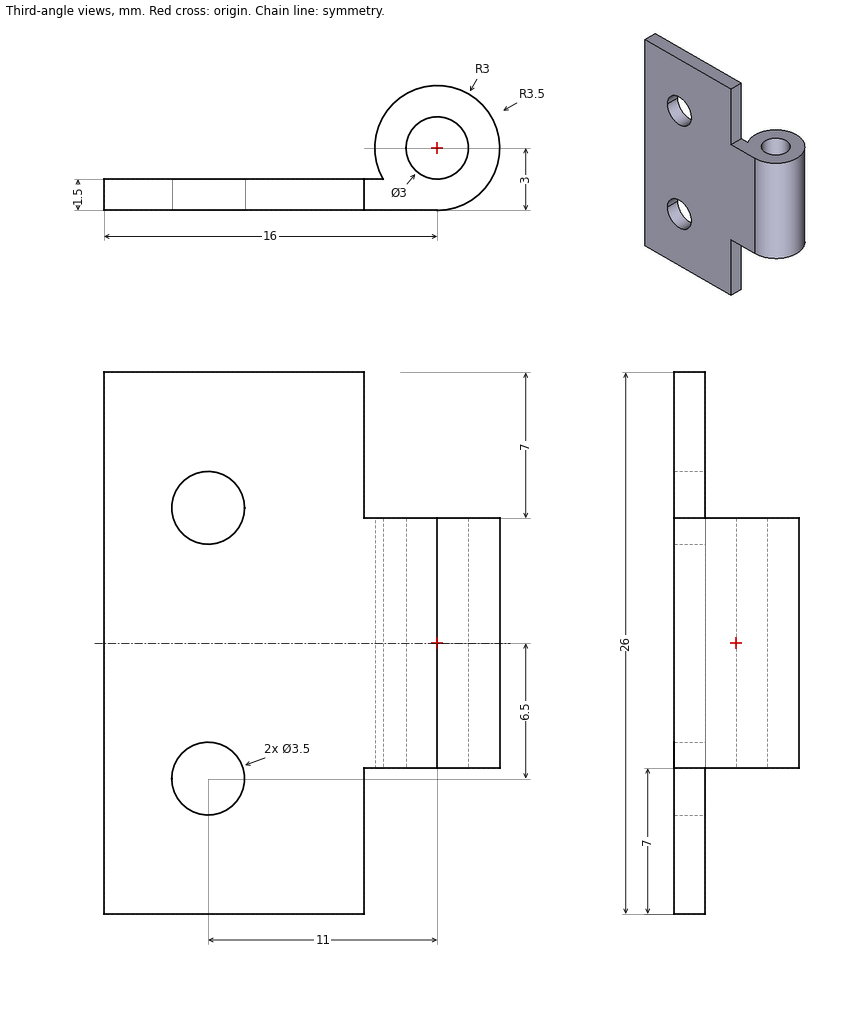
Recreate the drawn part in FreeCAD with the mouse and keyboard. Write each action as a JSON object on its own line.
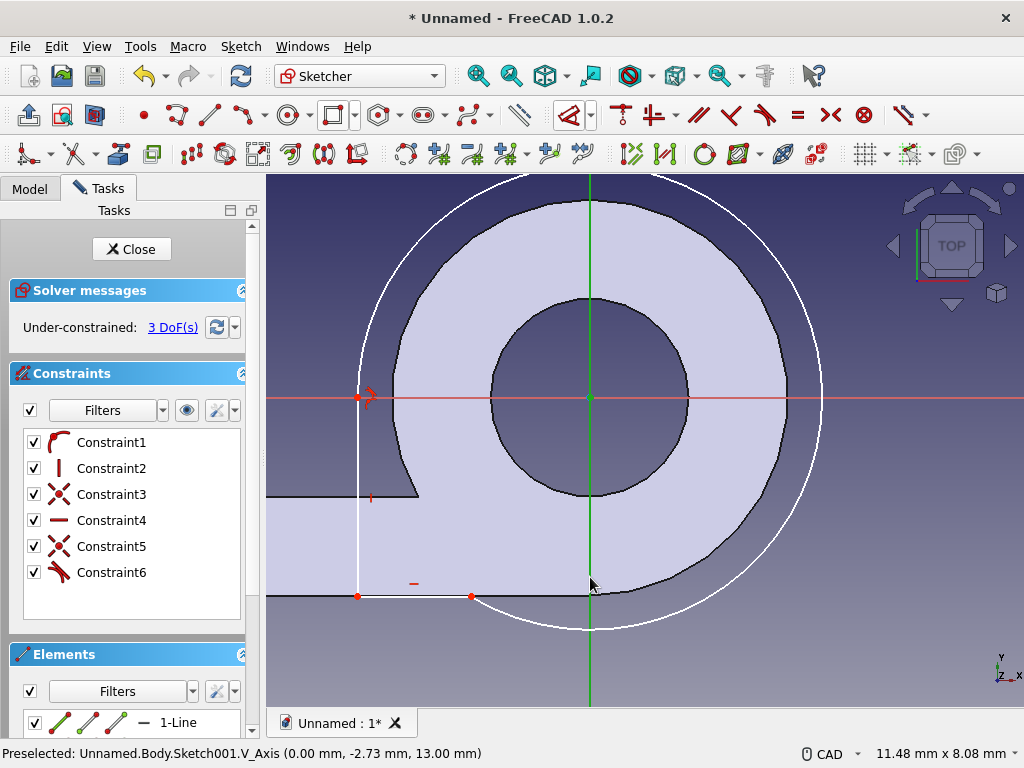
{"action": "left_click", "coordinate": [621, 116]}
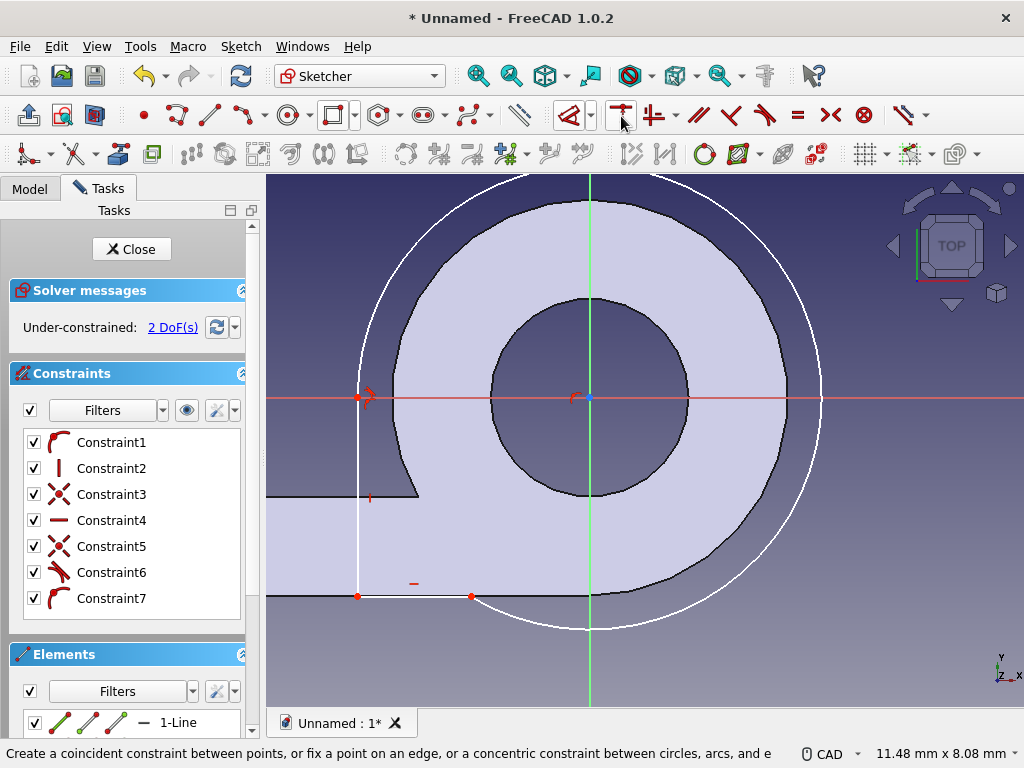
{"action": "left_click", "coordinate": [790, 516]}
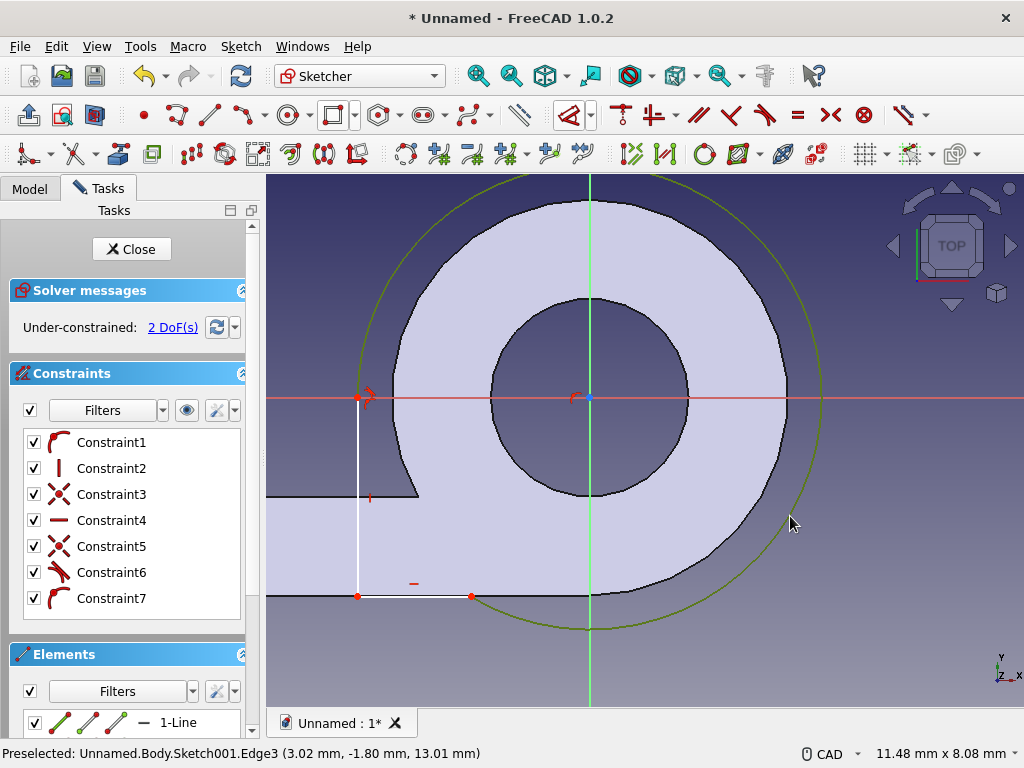
{"action": "left_click", "coordinate": [590, 116]}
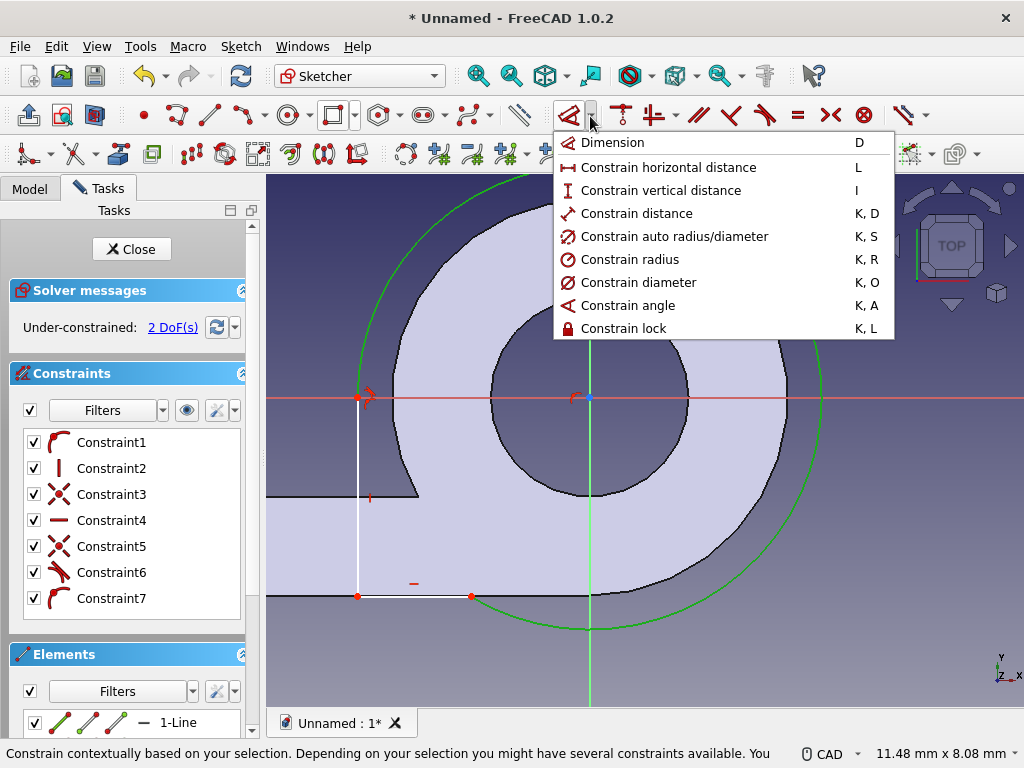
{"action": "left_click", "coordinate": [724, 260]}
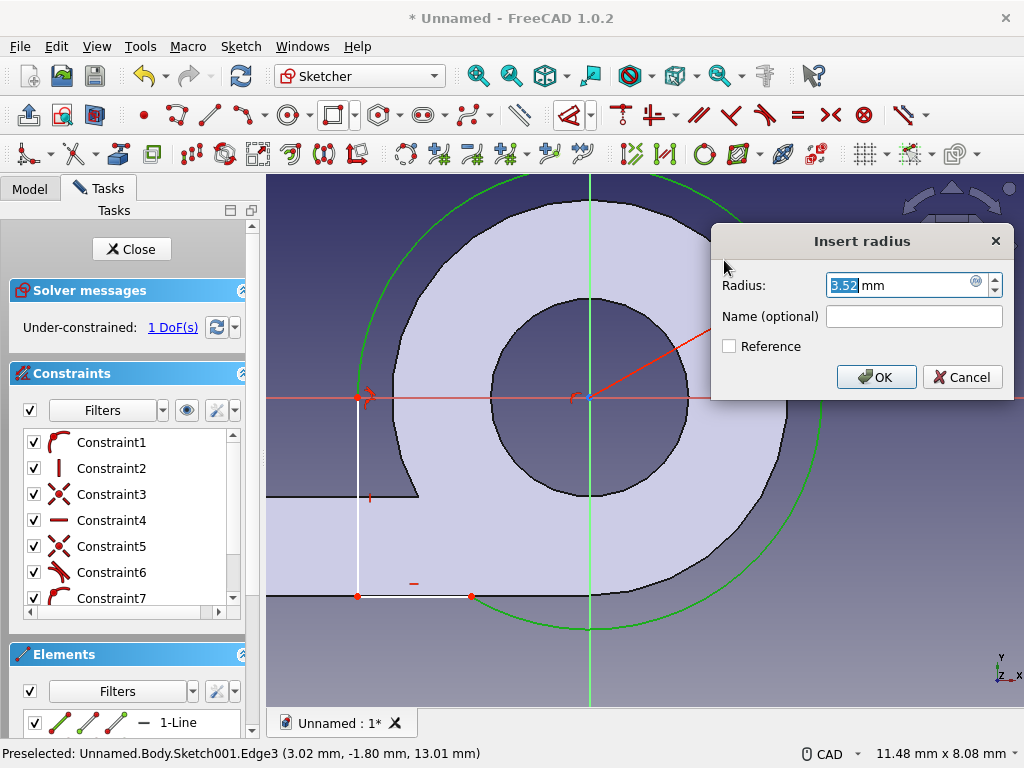
{"action": "type", "text": "3.5"}
{"action": "key", "text": "Return"}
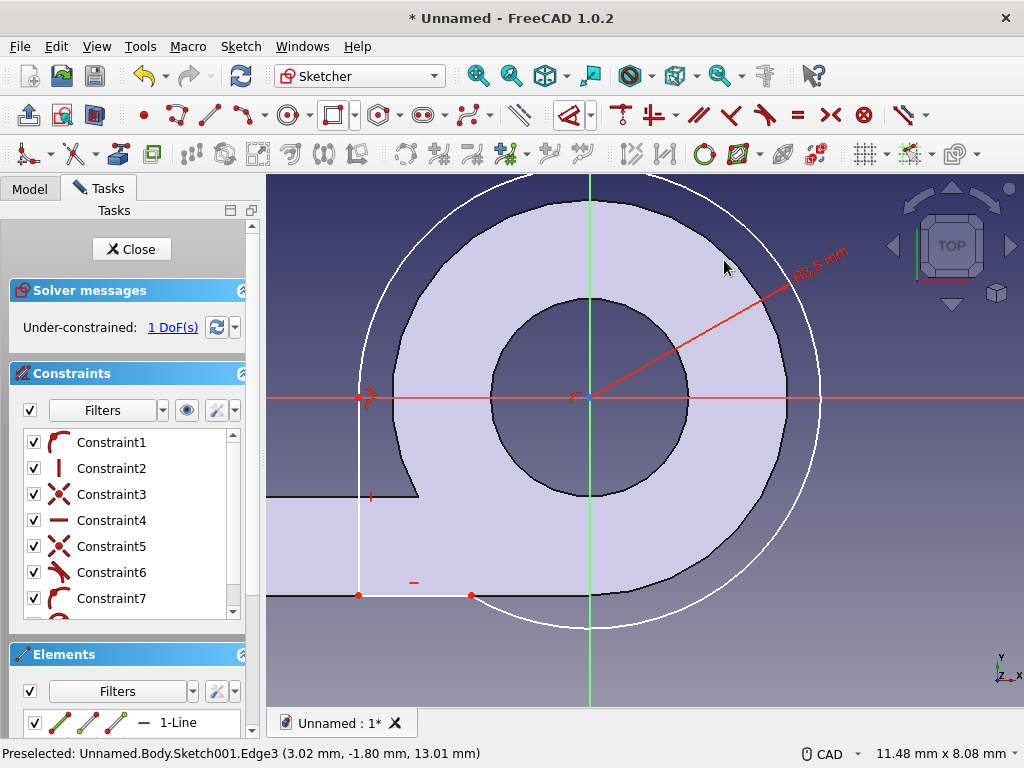
{"action": "left_click", "coordinate": [359, 457]}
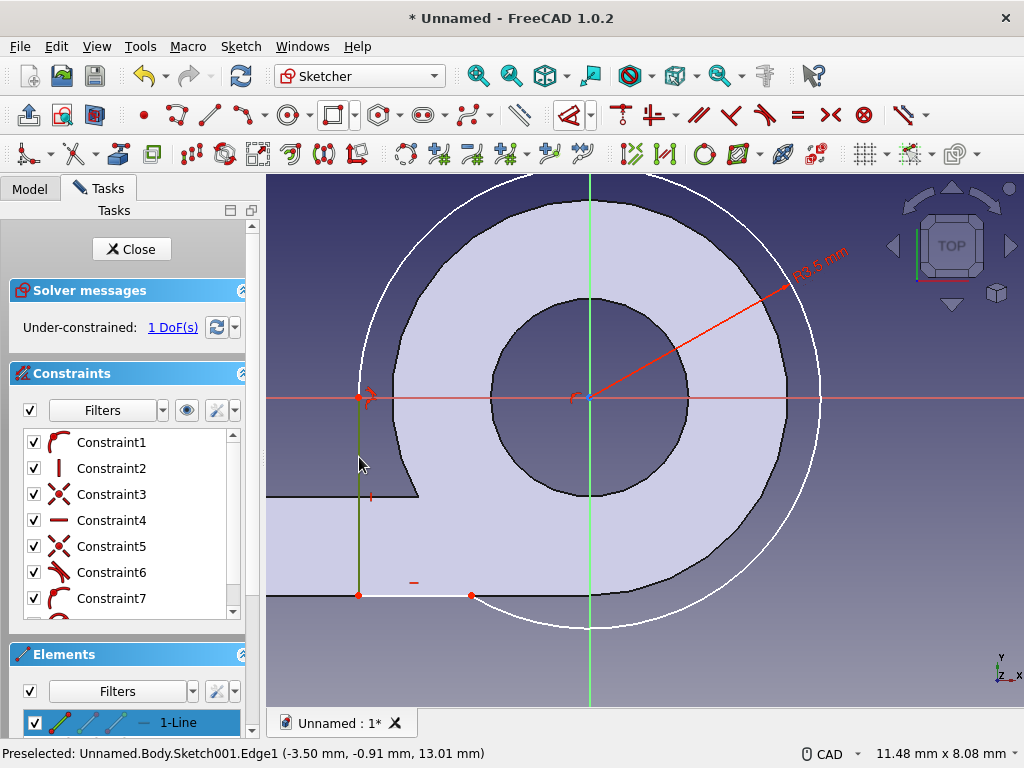
{"action": "key", "text": "i"}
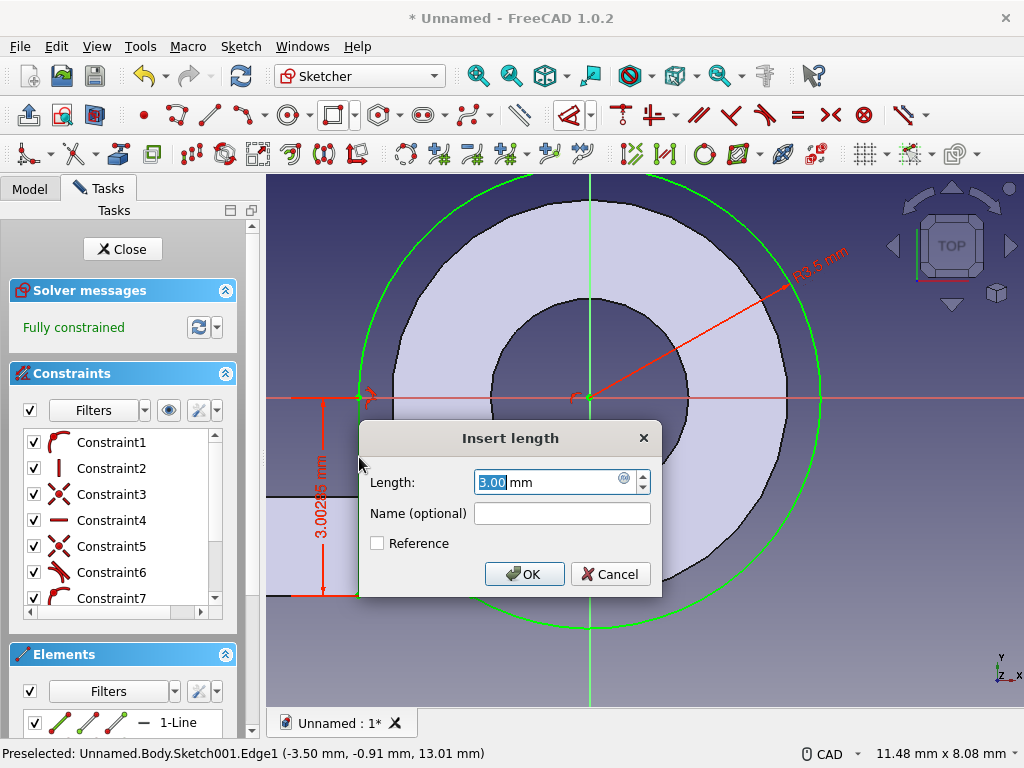
{"action": "type", "text": "3"}
{"action": "key", "text": "Return"}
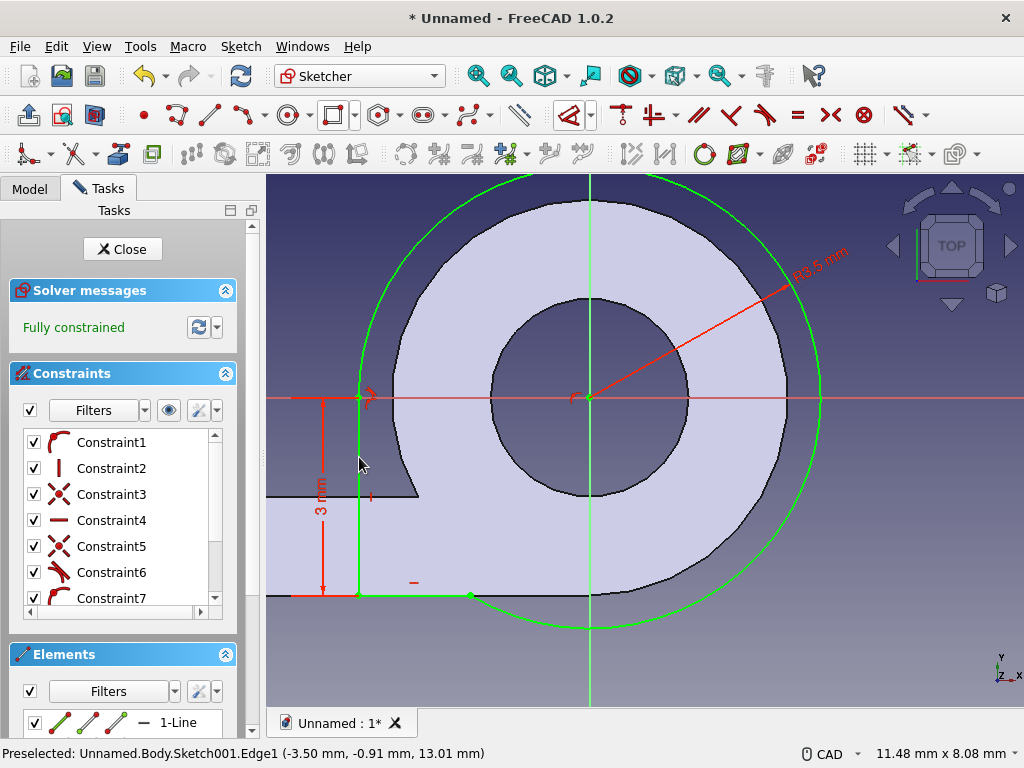
{"action": "left_click", "coordinate": [123, 249]}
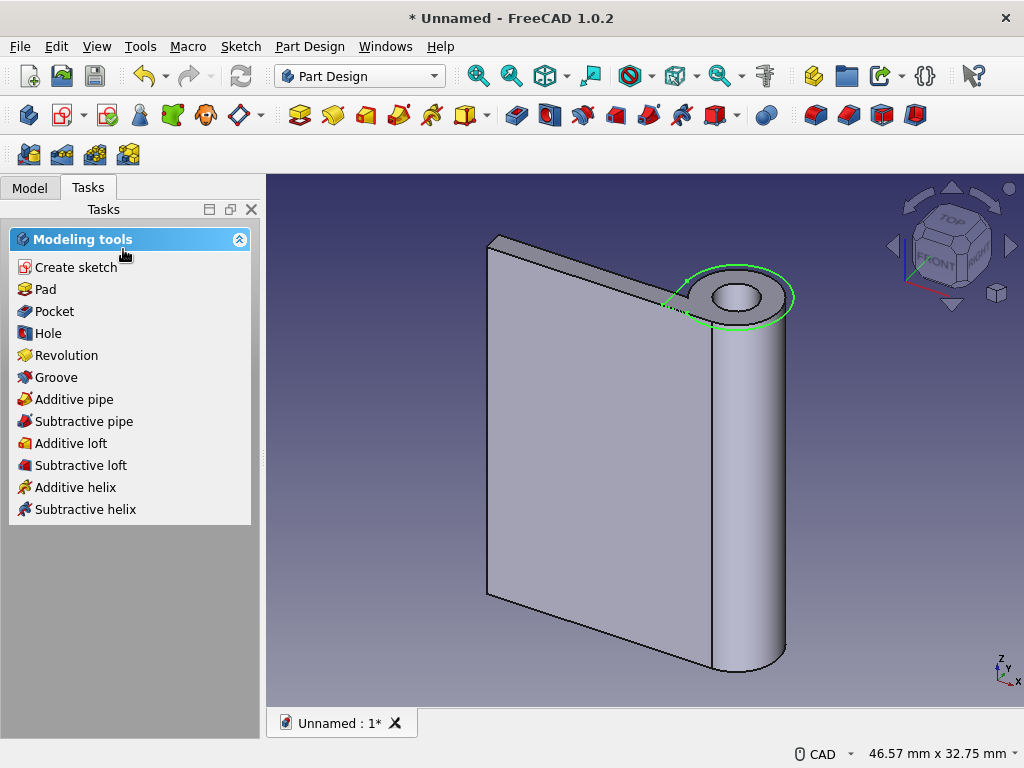
{"action": "left_click", "coordinate": [517, 116]}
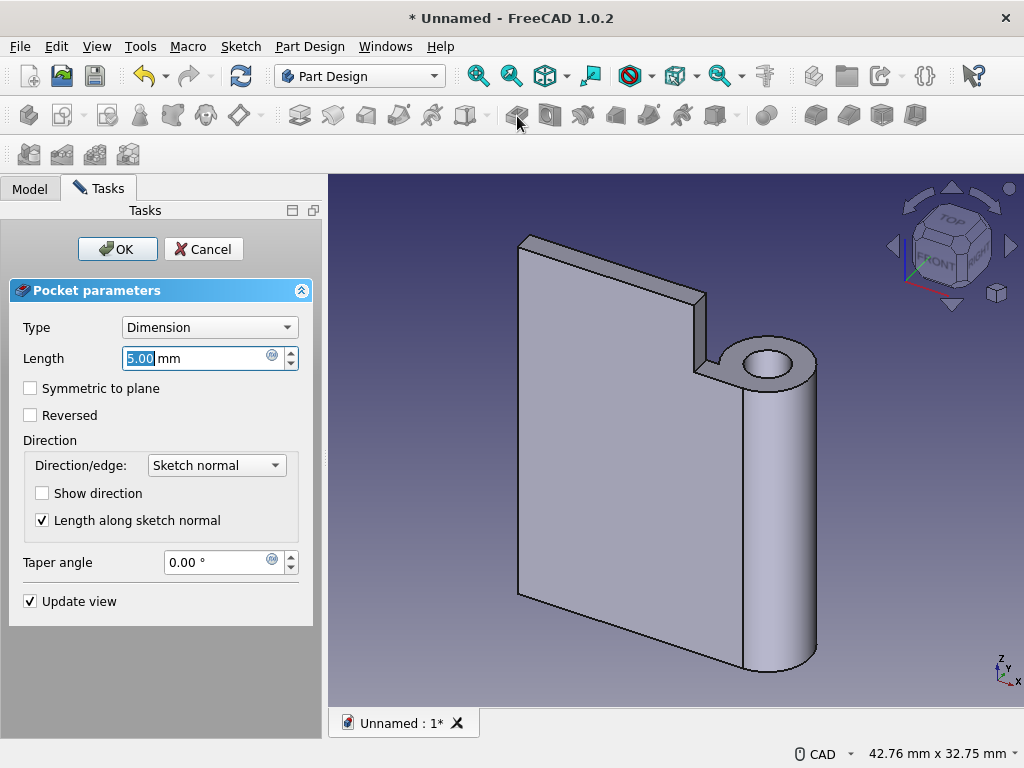
{"action": "type", "text": "7"}
{"action": "key", "text": "Tab"}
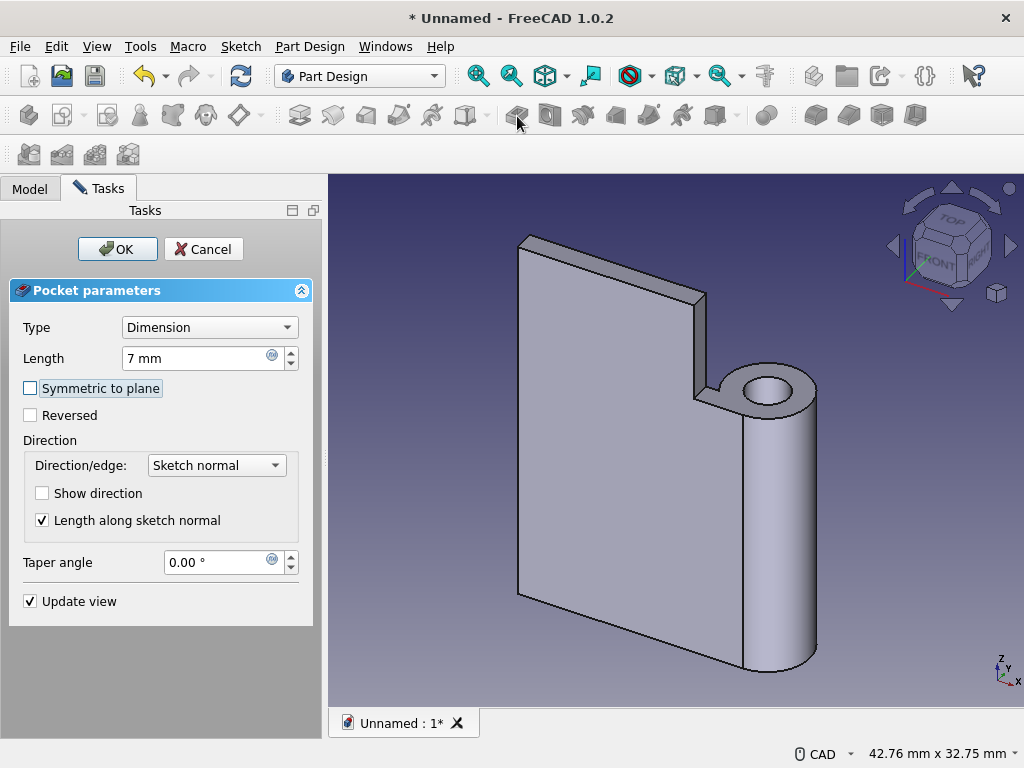
{"action": "left_click", "coordinate": [118, 249]}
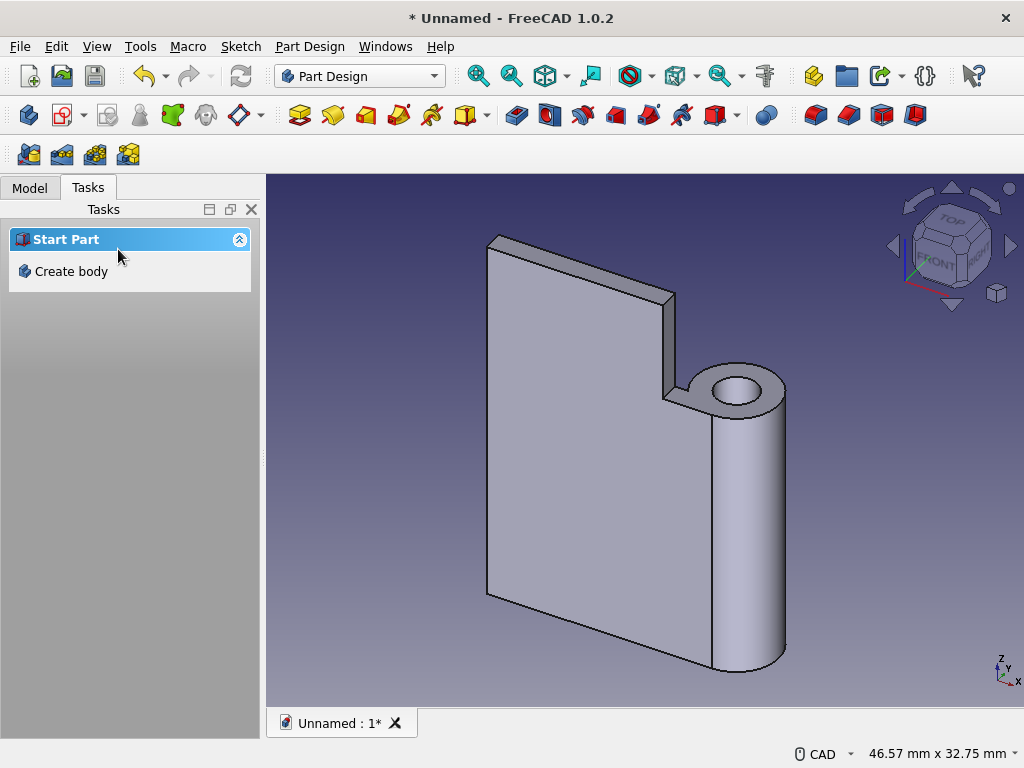
{"action": "key", "text": "5"}